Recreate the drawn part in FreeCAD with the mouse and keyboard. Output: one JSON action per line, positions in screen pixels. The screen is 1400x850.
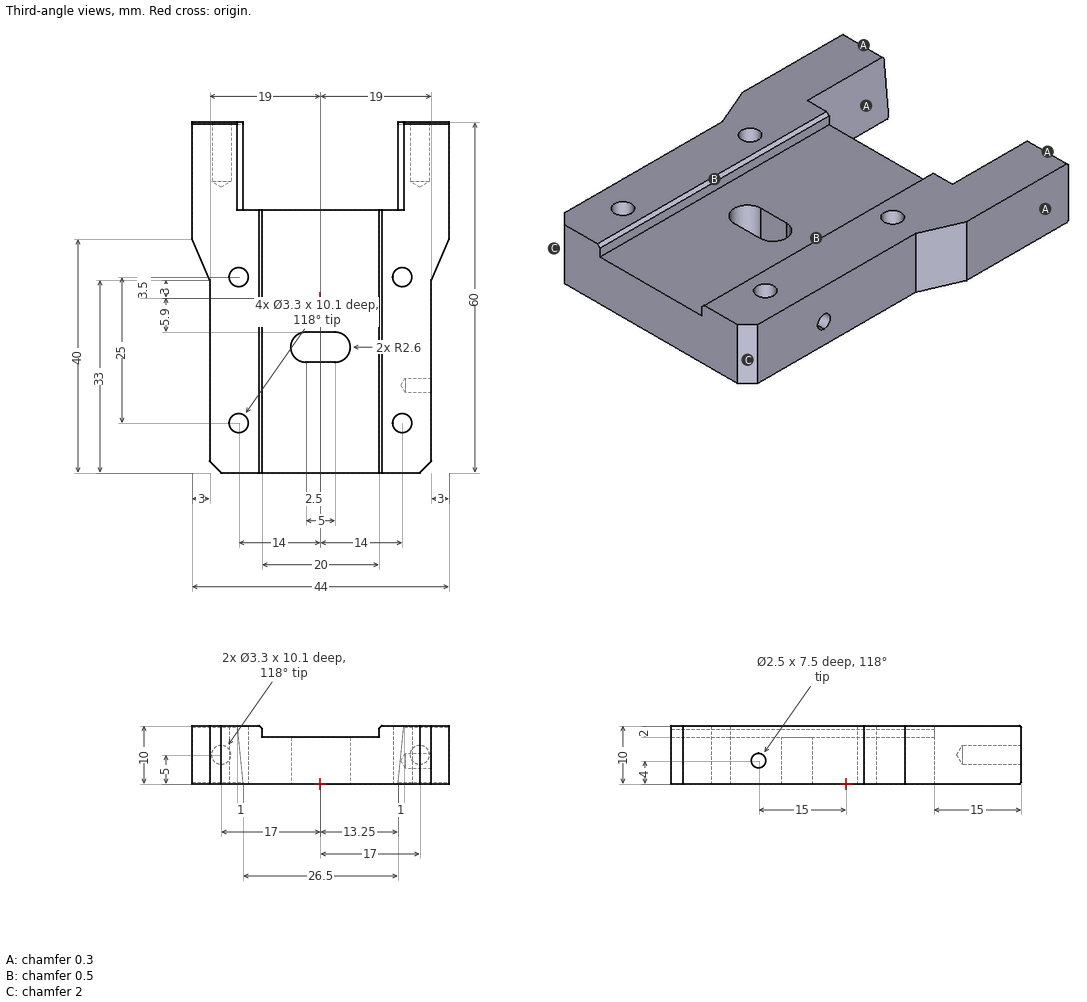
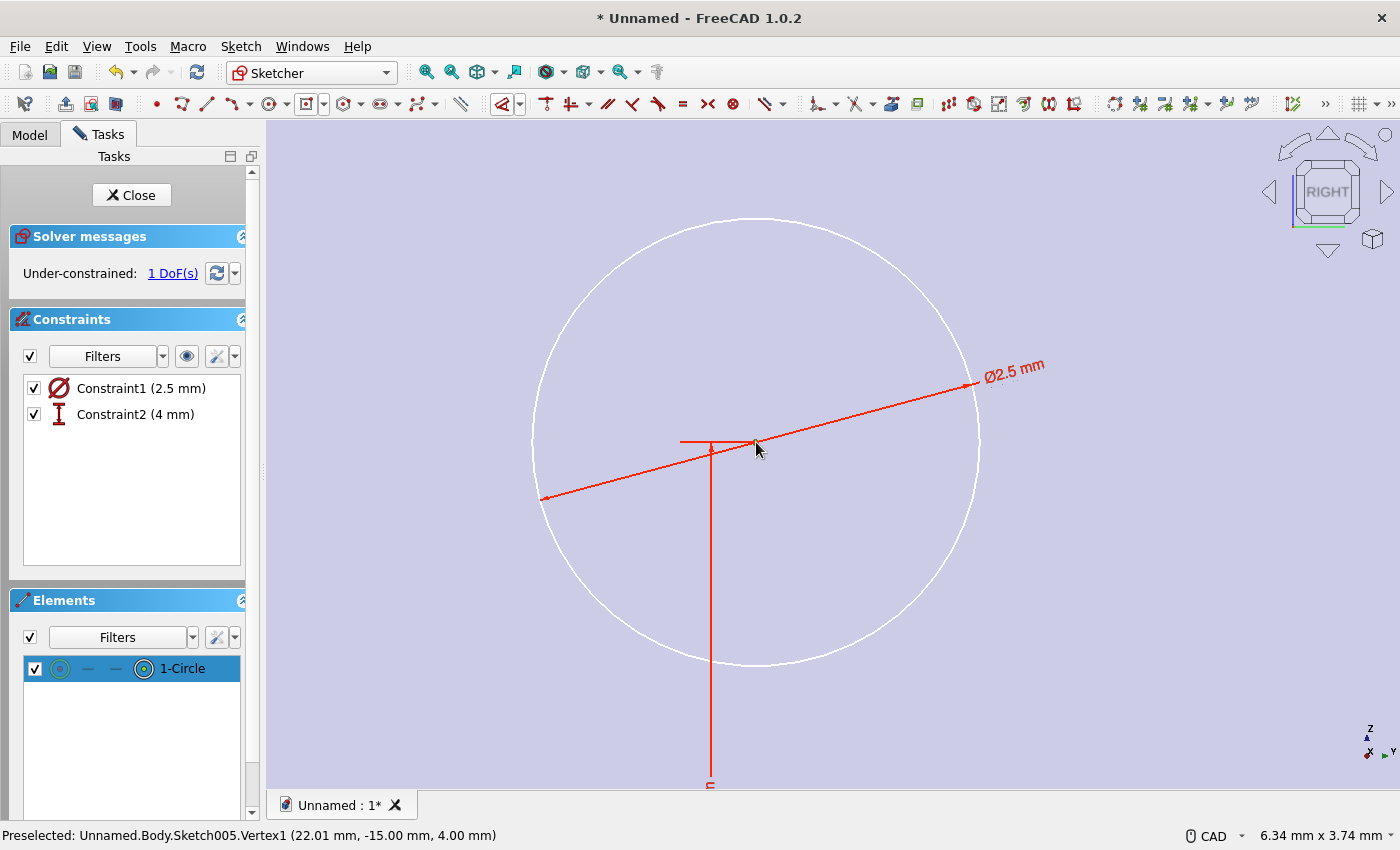
{"action": "left_click", "coordinate": [520, 104]}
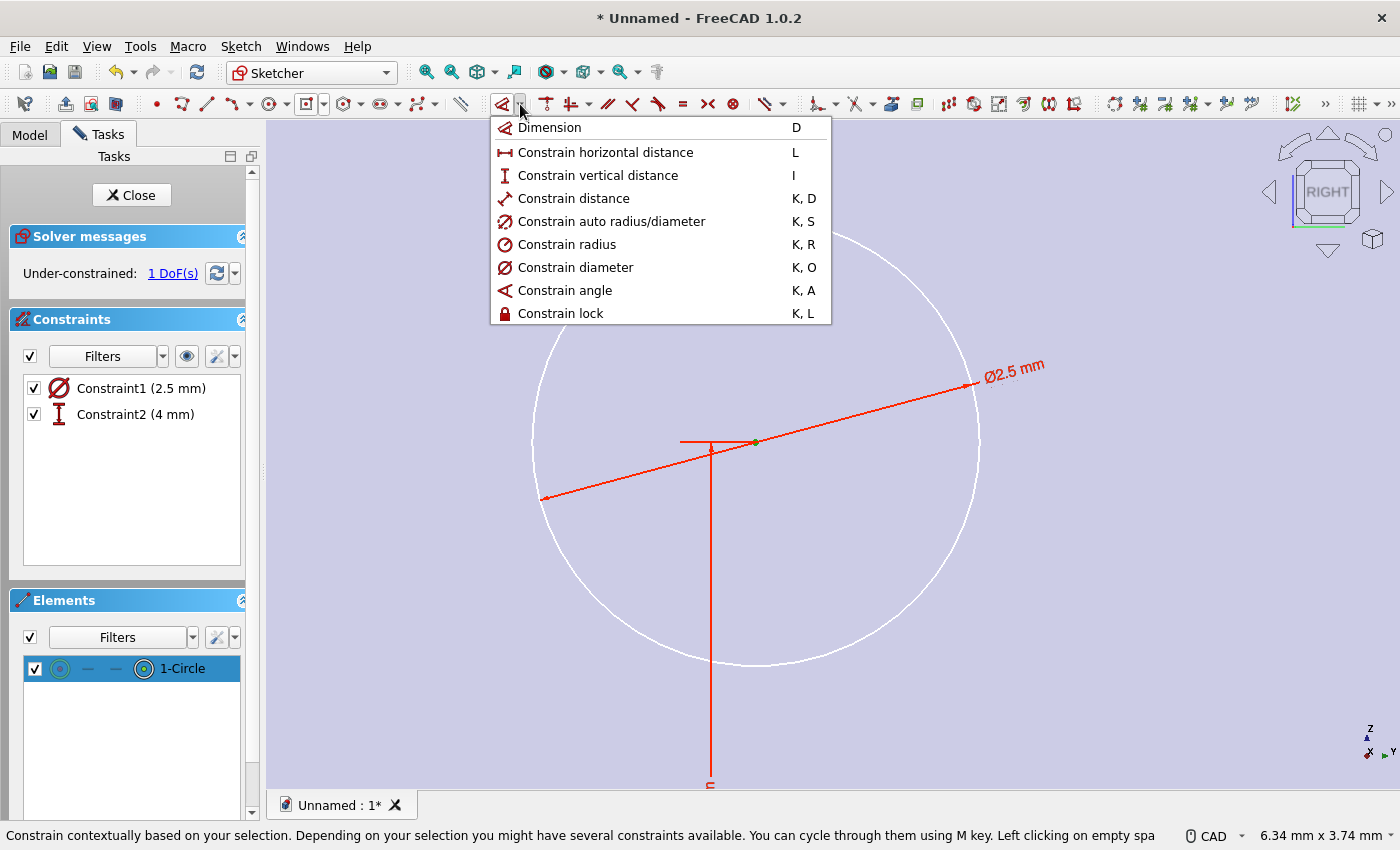
{"action": "left_click", "coordinate": [661, 152]}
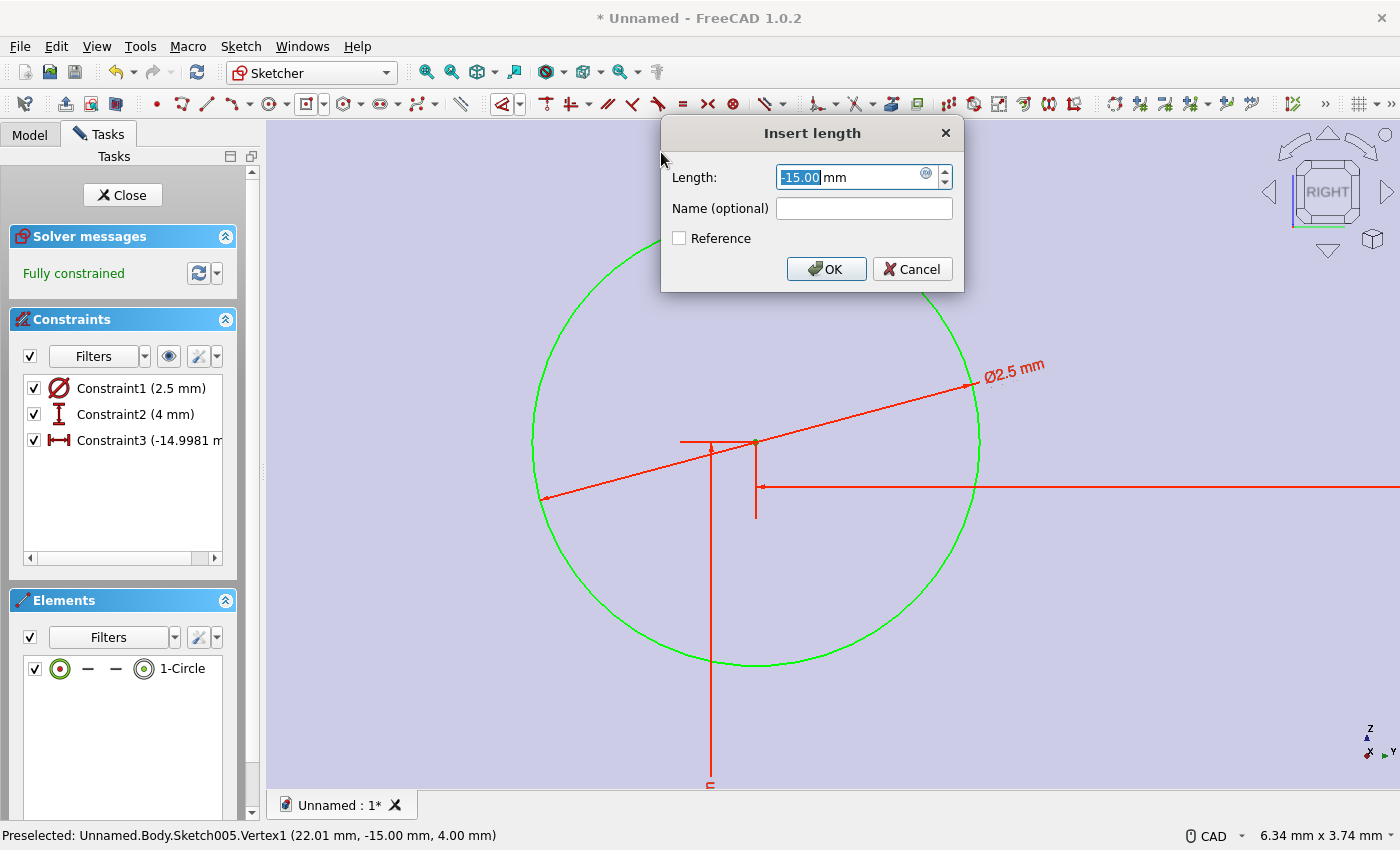
{"action": "type", "text": "-15"}
{"action": "key", "text": "Return"}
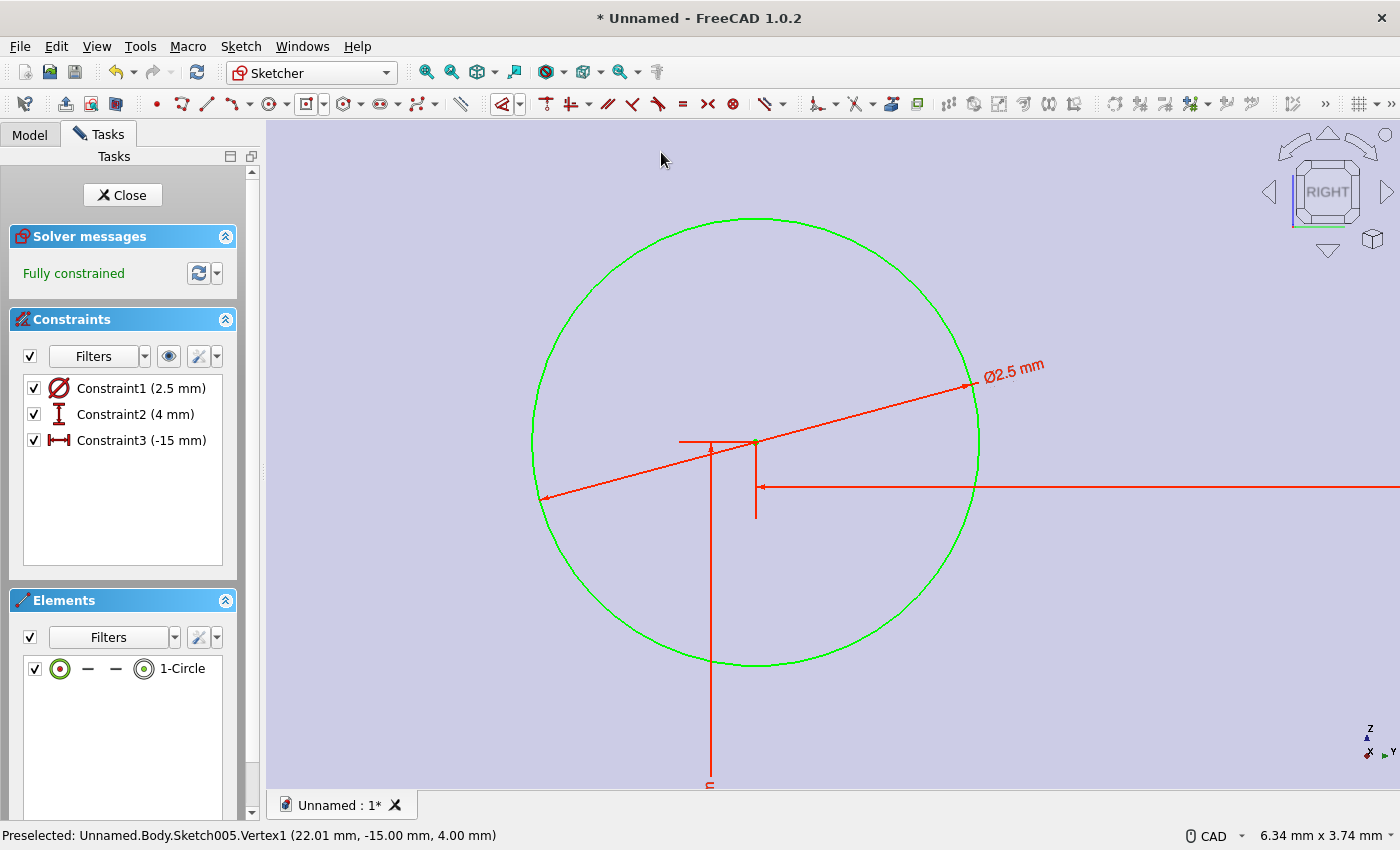
{"action": "left_click", "coordinate": [123, 195]}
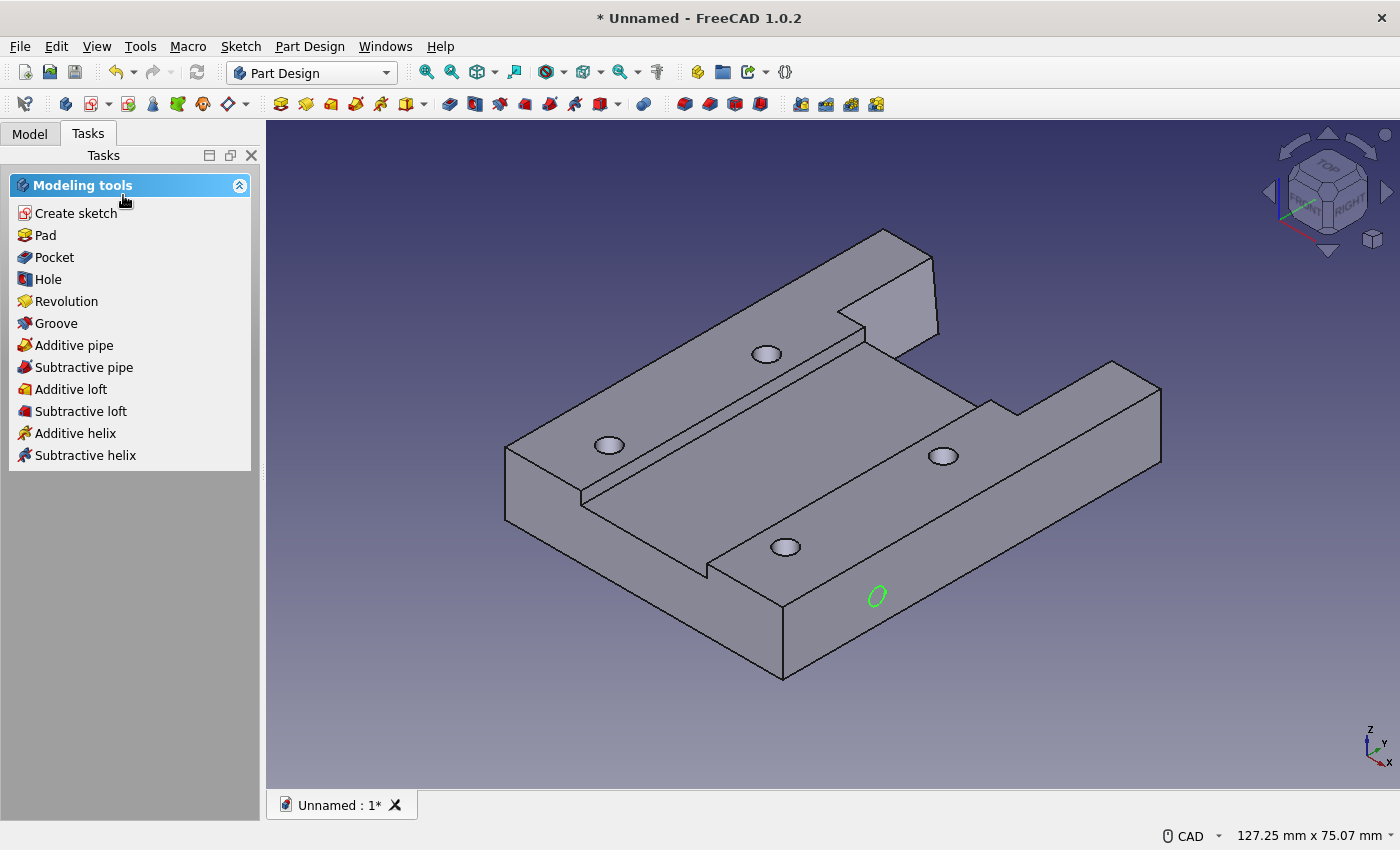
{"action": "left_click", "coordinate": [475, 104]}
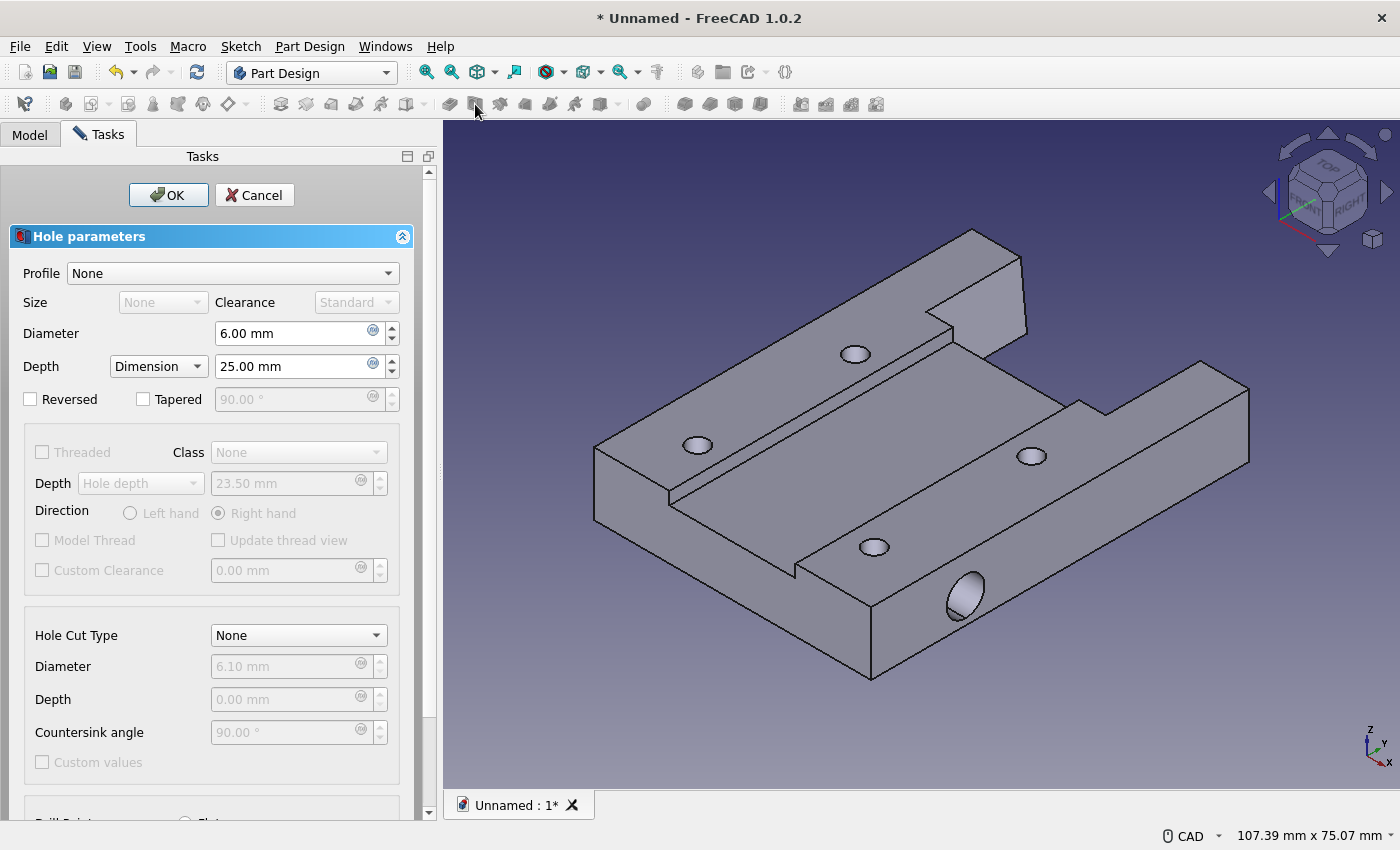
{"action": "triple_click", "coordinate": [300, 334]}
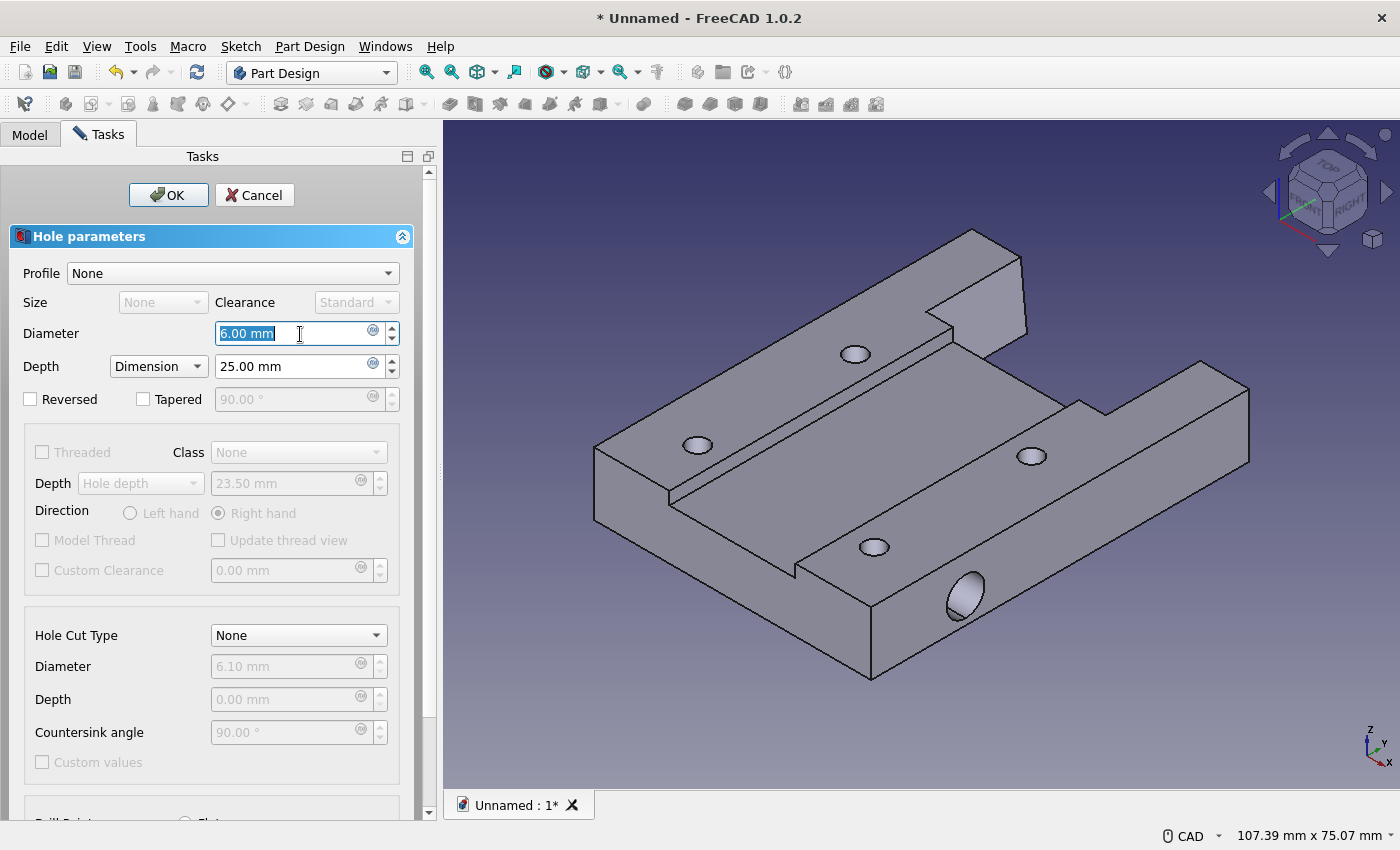
{"action": "type", "text": "2.5"}
{"action": "key", "text": "Tab"}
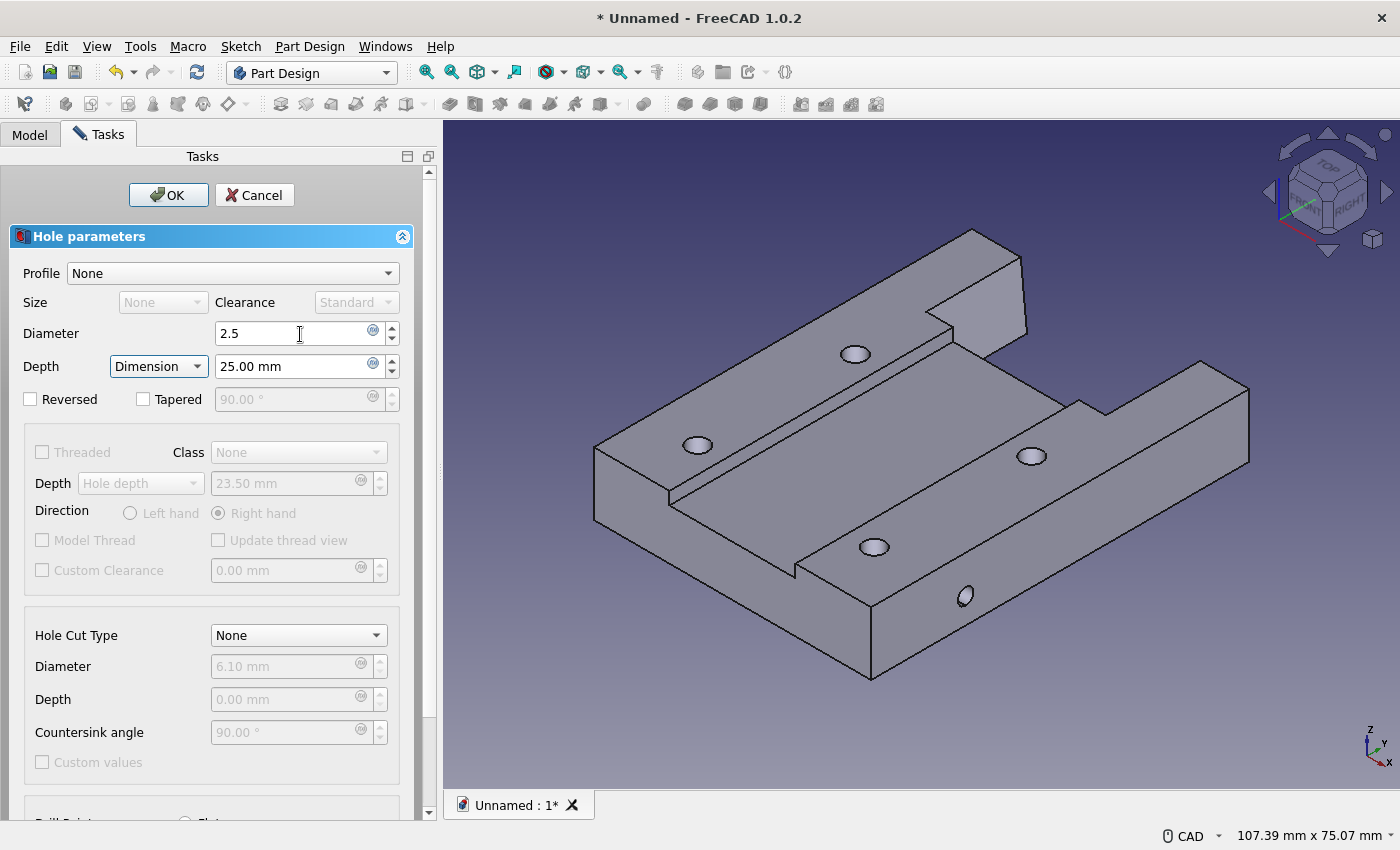
{"action": "triple_click", "coordinate": [300, 366]}